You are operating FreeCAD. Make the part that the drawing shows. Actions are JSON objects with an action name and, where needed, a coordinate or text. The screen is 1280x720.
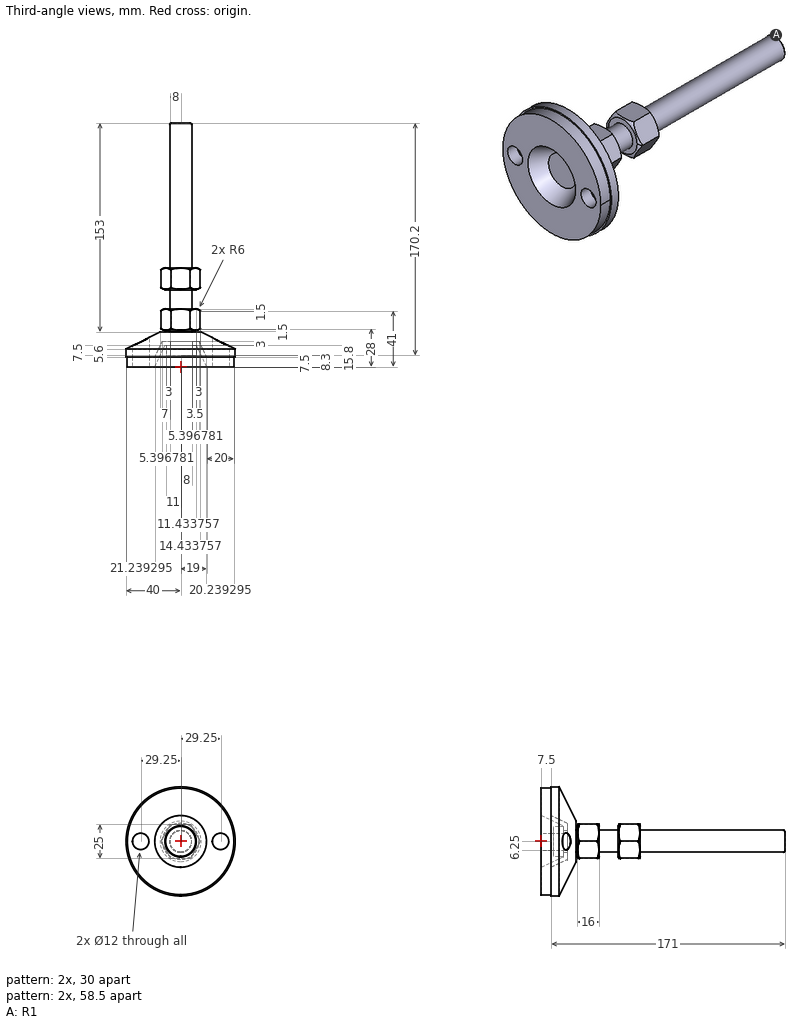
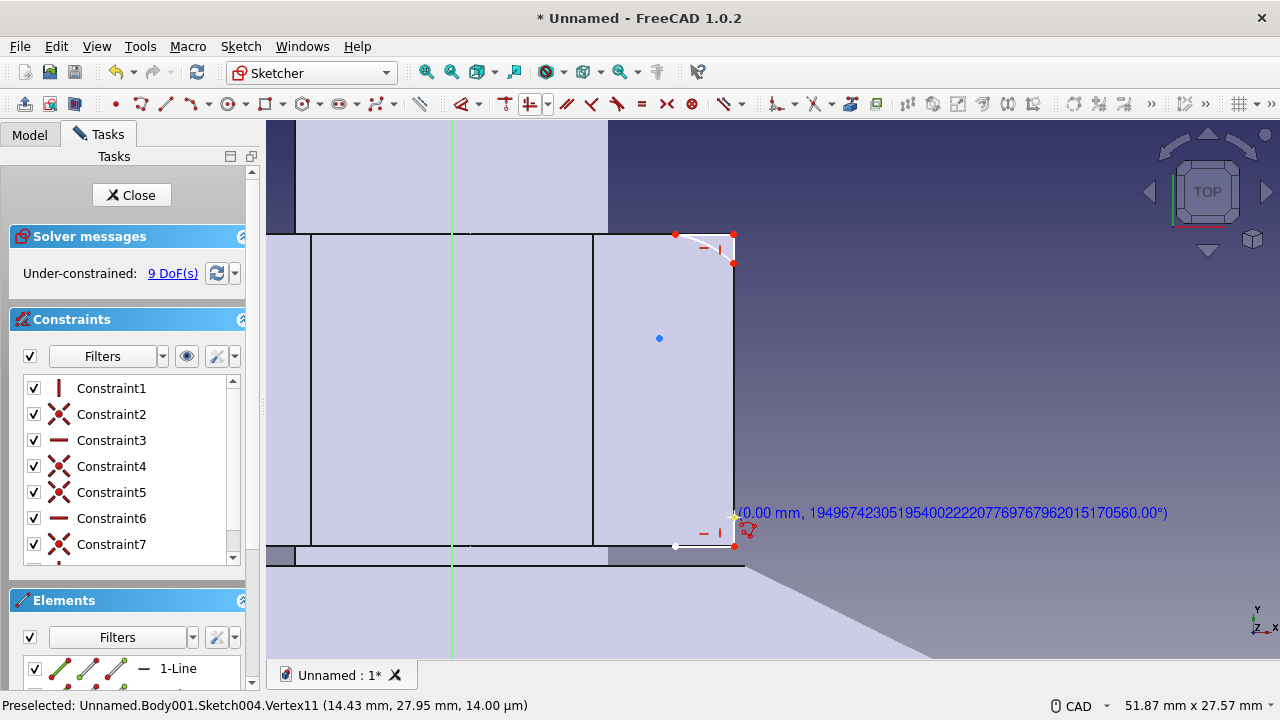
{"action": "left_click", "coordinate": [190, 104]}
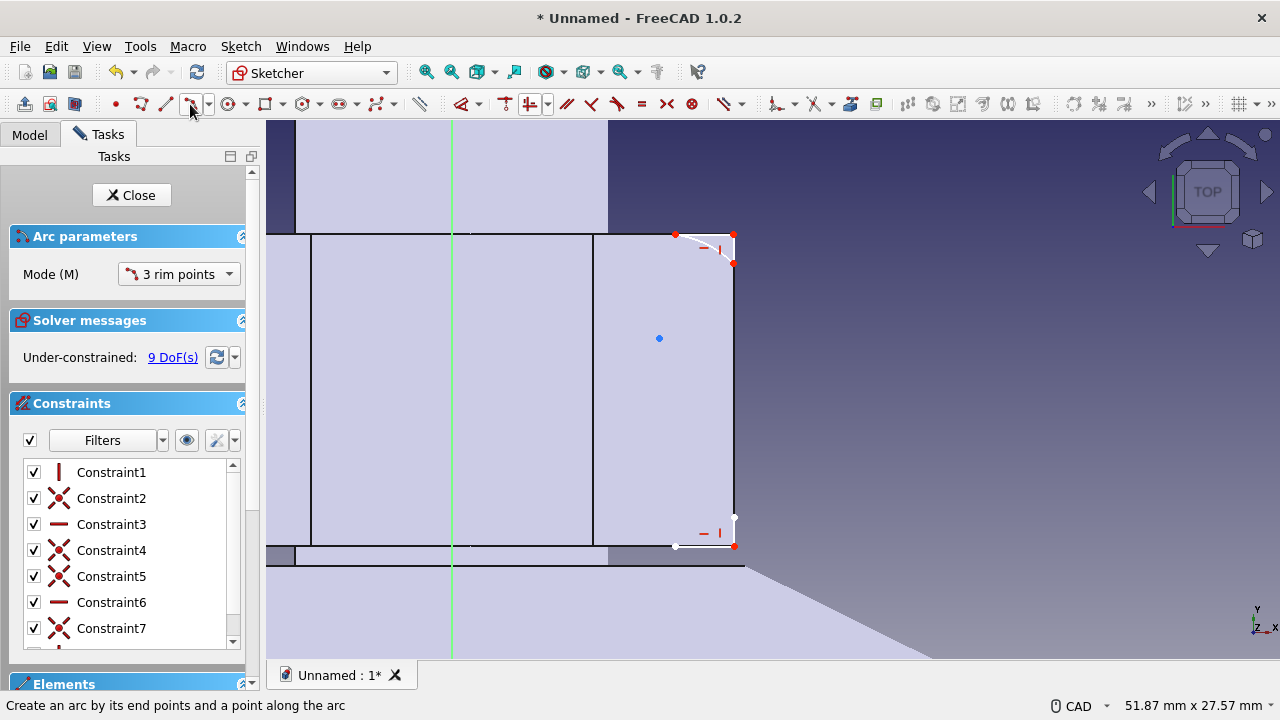
{"action": "left_click", "coordinate": [734, 518]}
{"action": "left_click", "coordinate": [675, 547]}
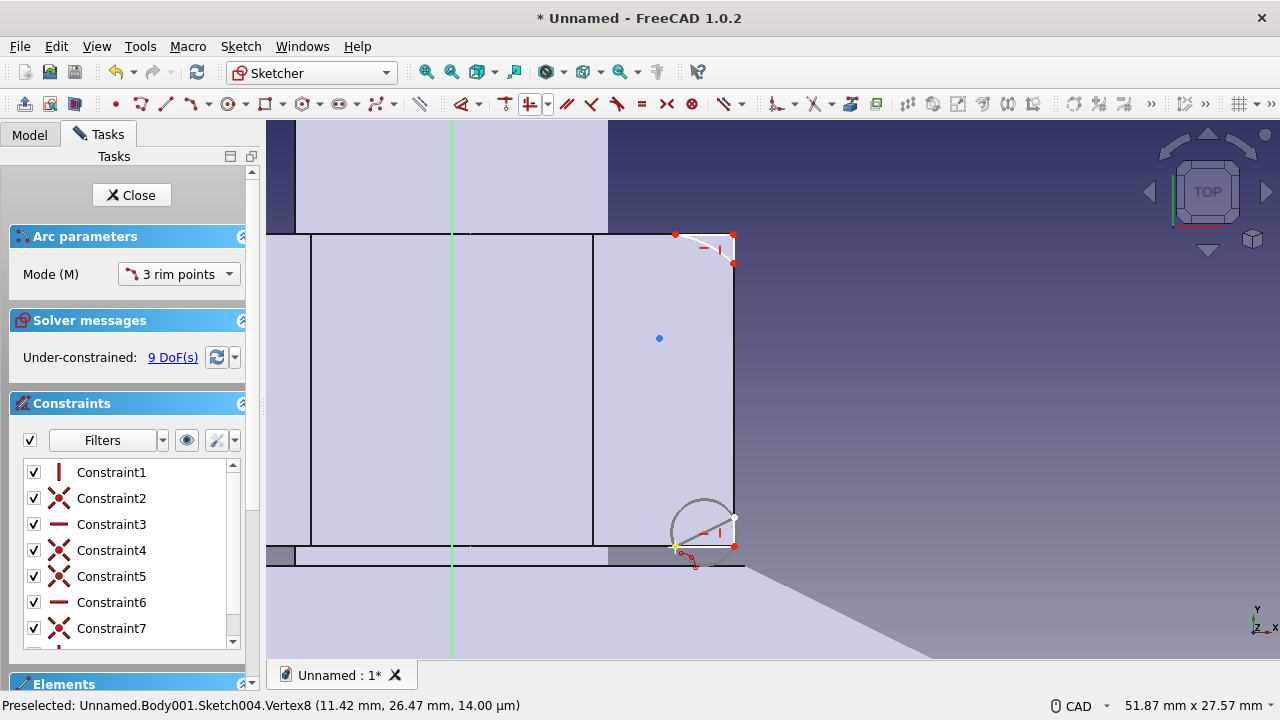
{"action": "scroll", "coordinate": [707, 536], "scroll_direction": "up", "scroll_amount": 7}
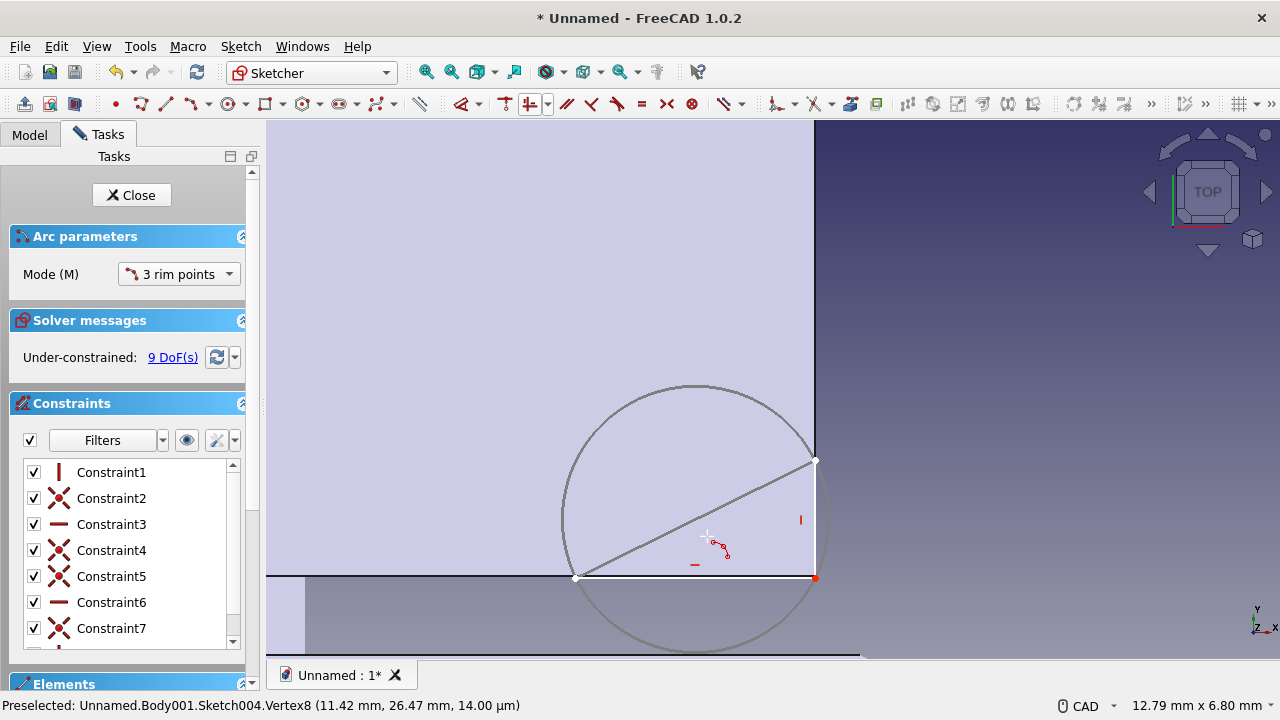
{"action": "left_click", "coordinate": [705, 533]}
{"action": "key", "text": "Escape"}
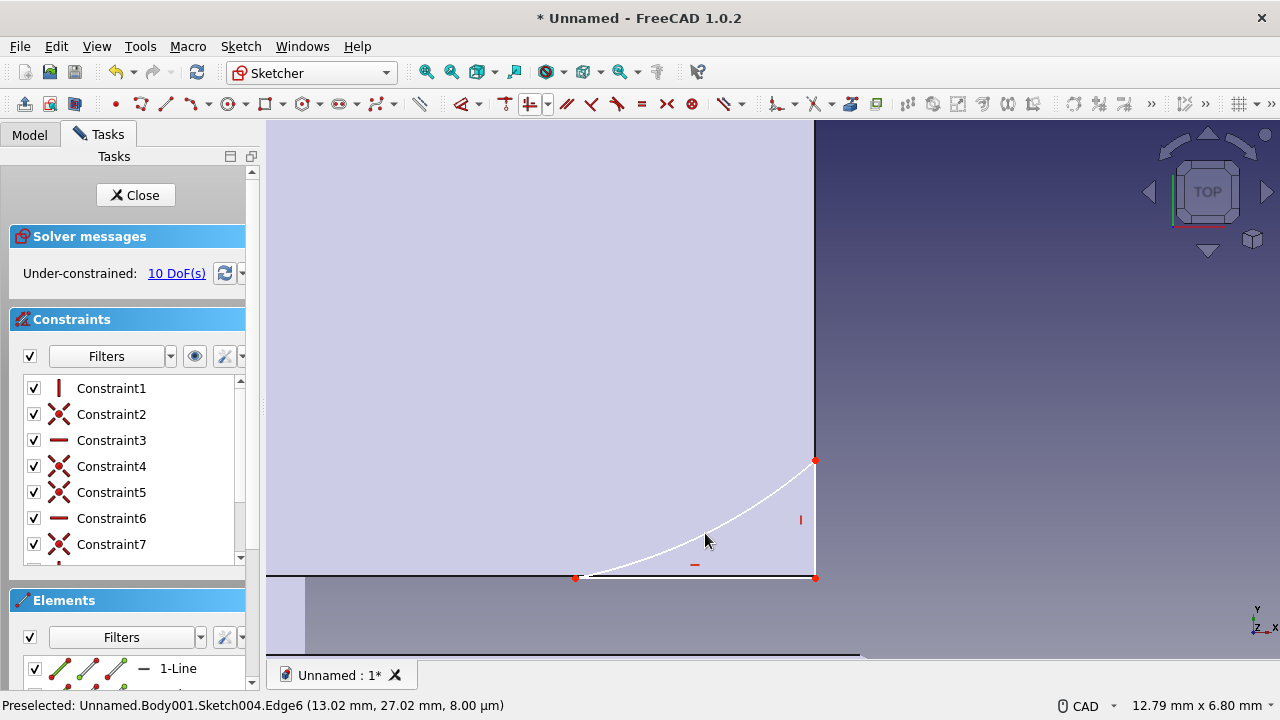
{"action": "scroll", "coordinate": [707, 536], "scroll_direction": "down", "scroll_amount": 7}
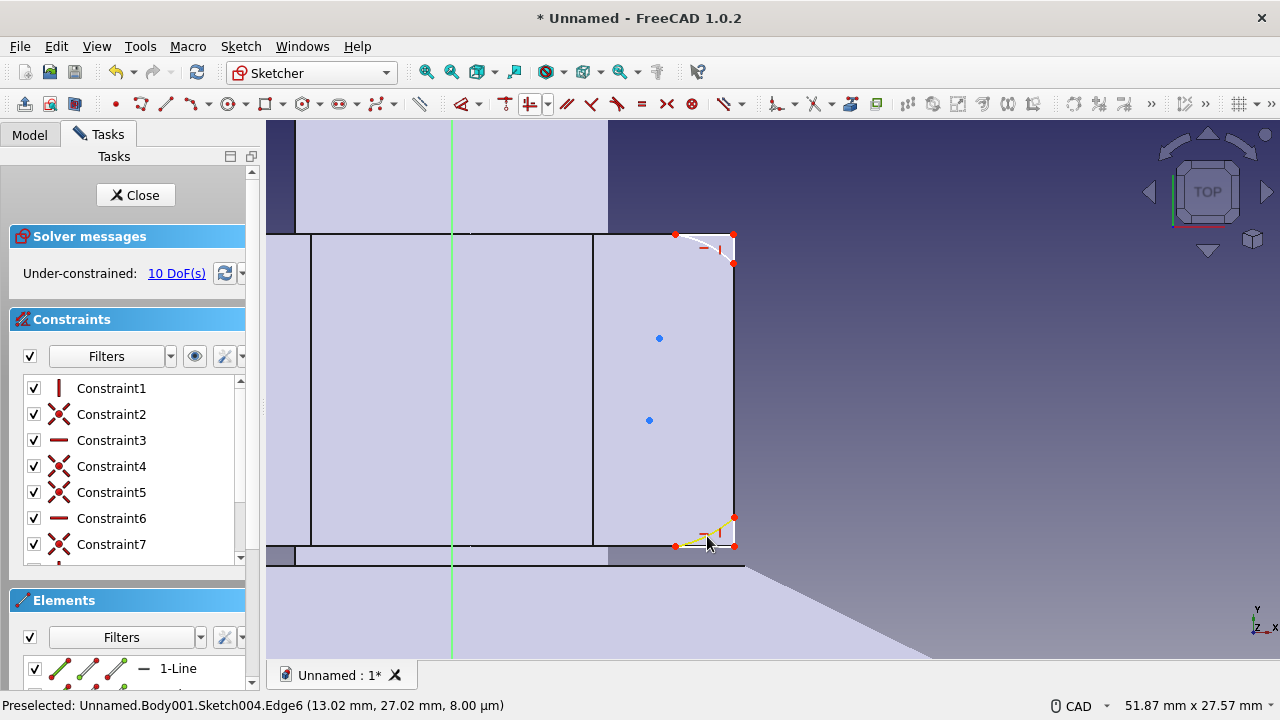
{"action": "left_click", "coordinate": [695, 239]}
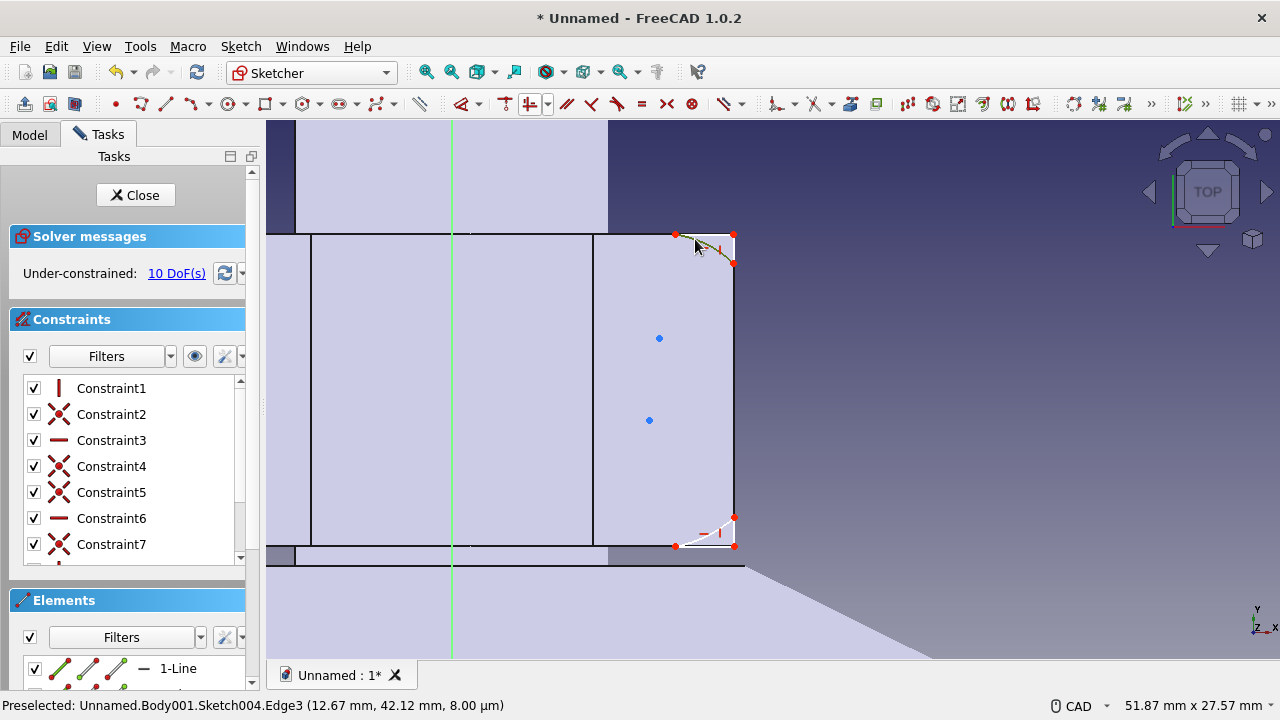
{"action": "scroll", "coordinate": [718, 530], "scroll_direction": "up", "scroll_amount": 4}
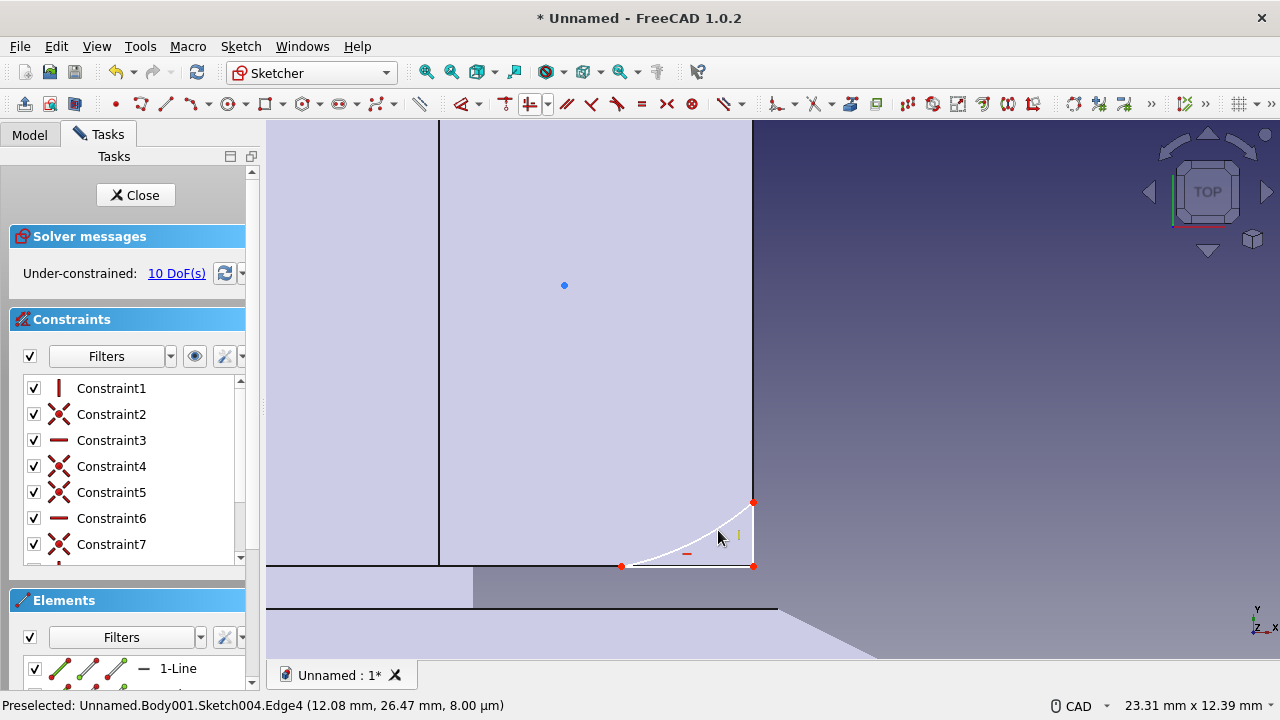
{"action": "left_click", "coordinate": [717, 529]}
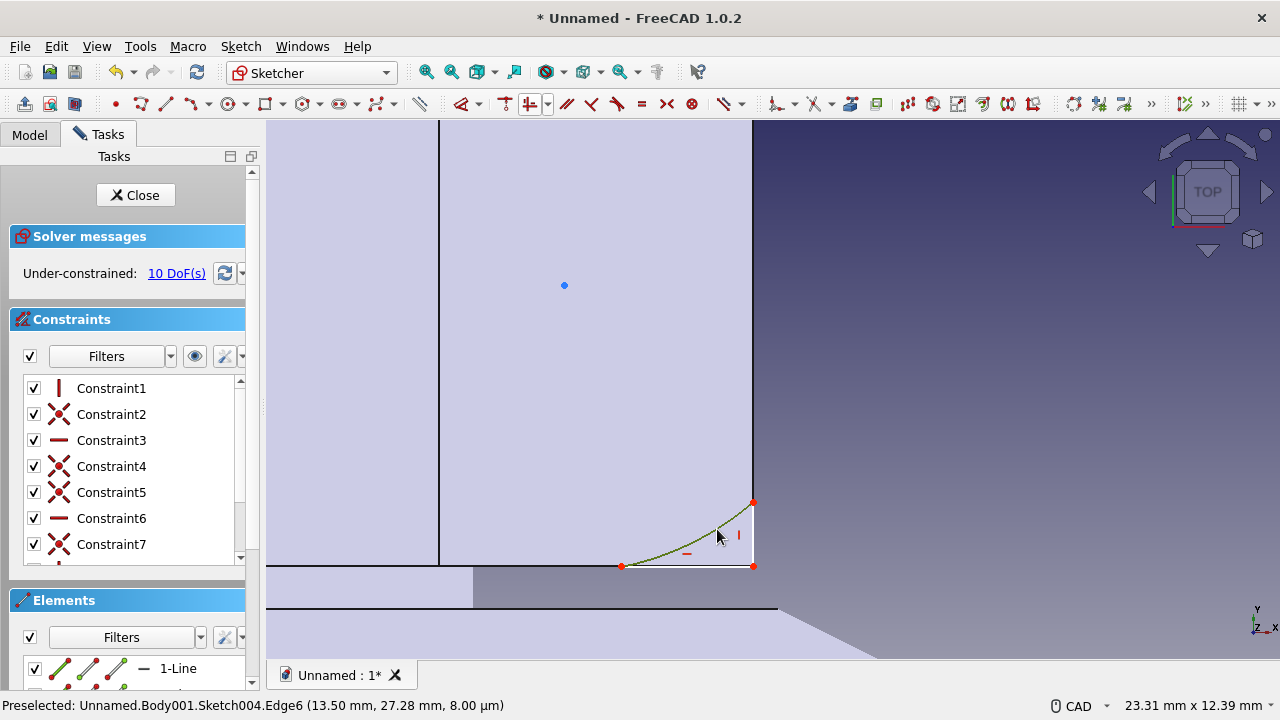
{"action": "left_click", "coordinate": [642, 104]}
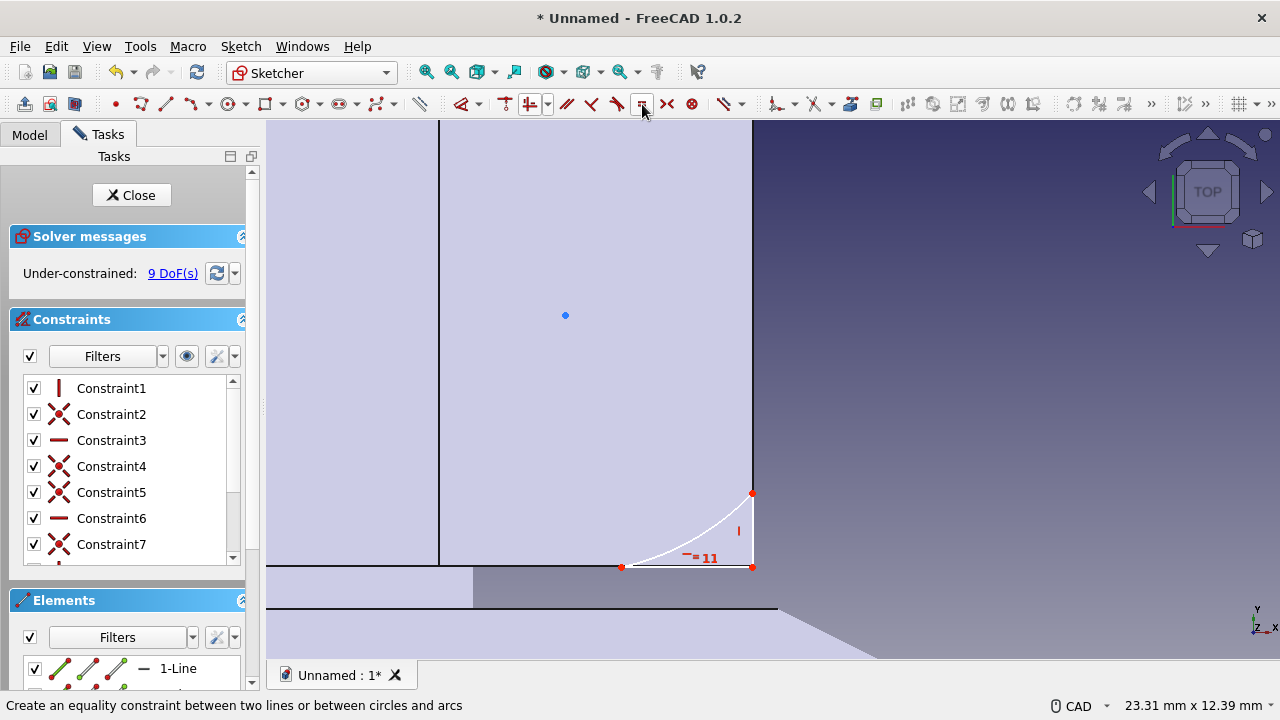
{"action": "left_click", "coordinate": [460, 104]}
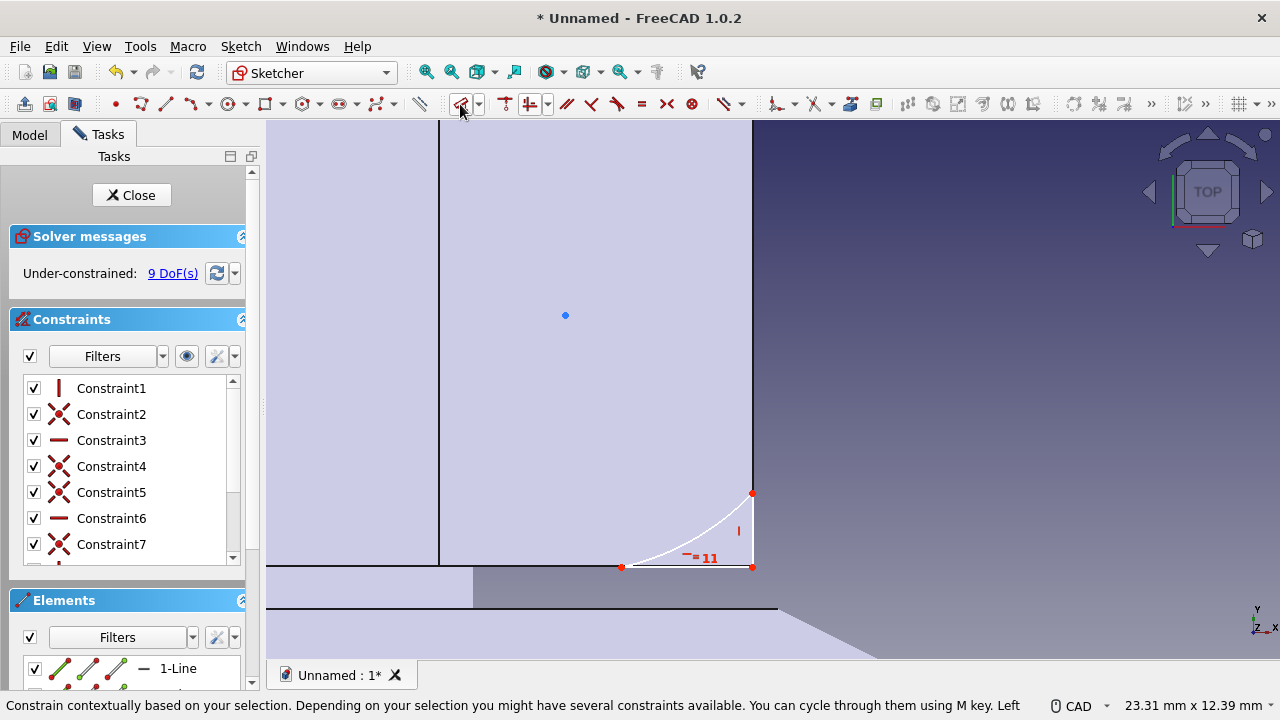
{"action": "scroll", "coordinate": [718, 530], "scroll_direction": "down", "scroll_amount": 4}